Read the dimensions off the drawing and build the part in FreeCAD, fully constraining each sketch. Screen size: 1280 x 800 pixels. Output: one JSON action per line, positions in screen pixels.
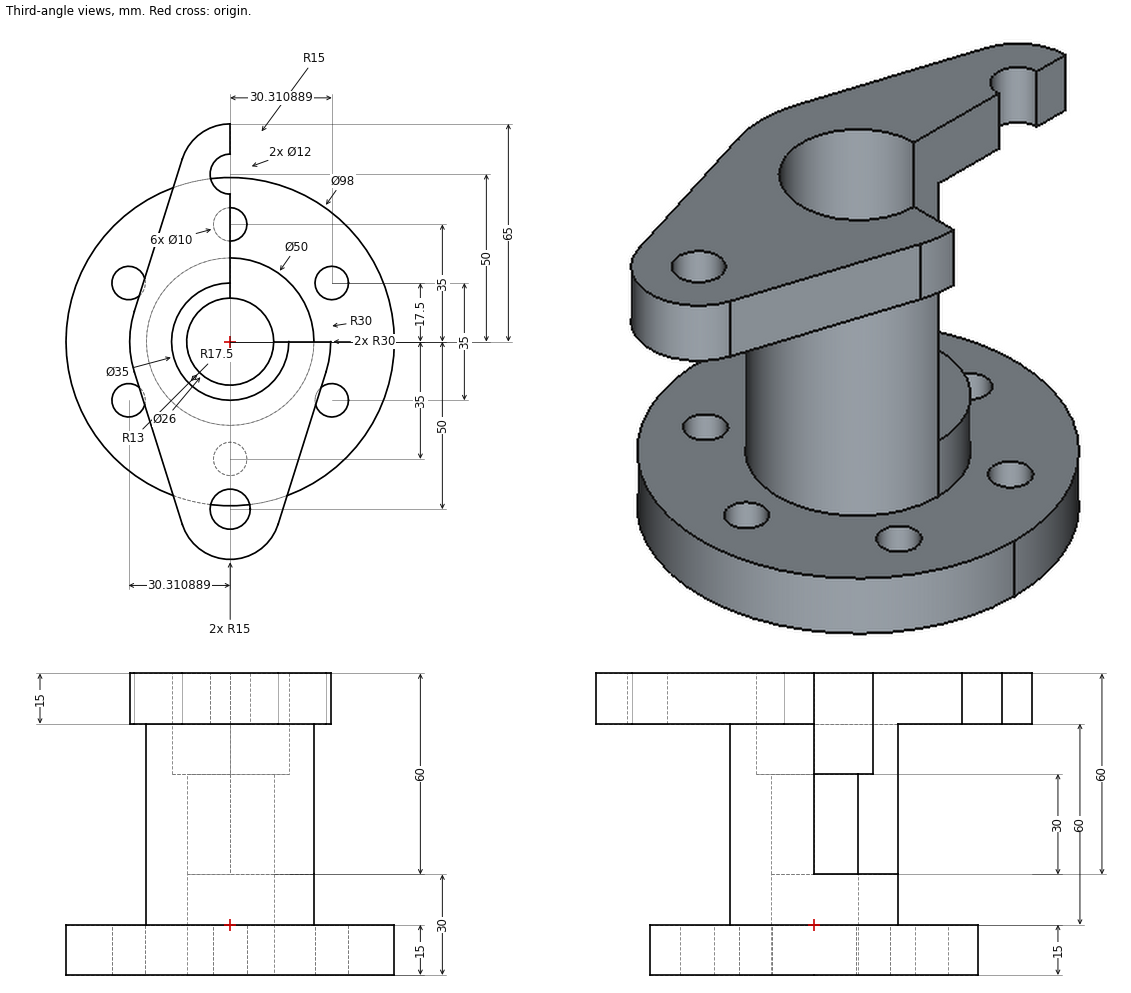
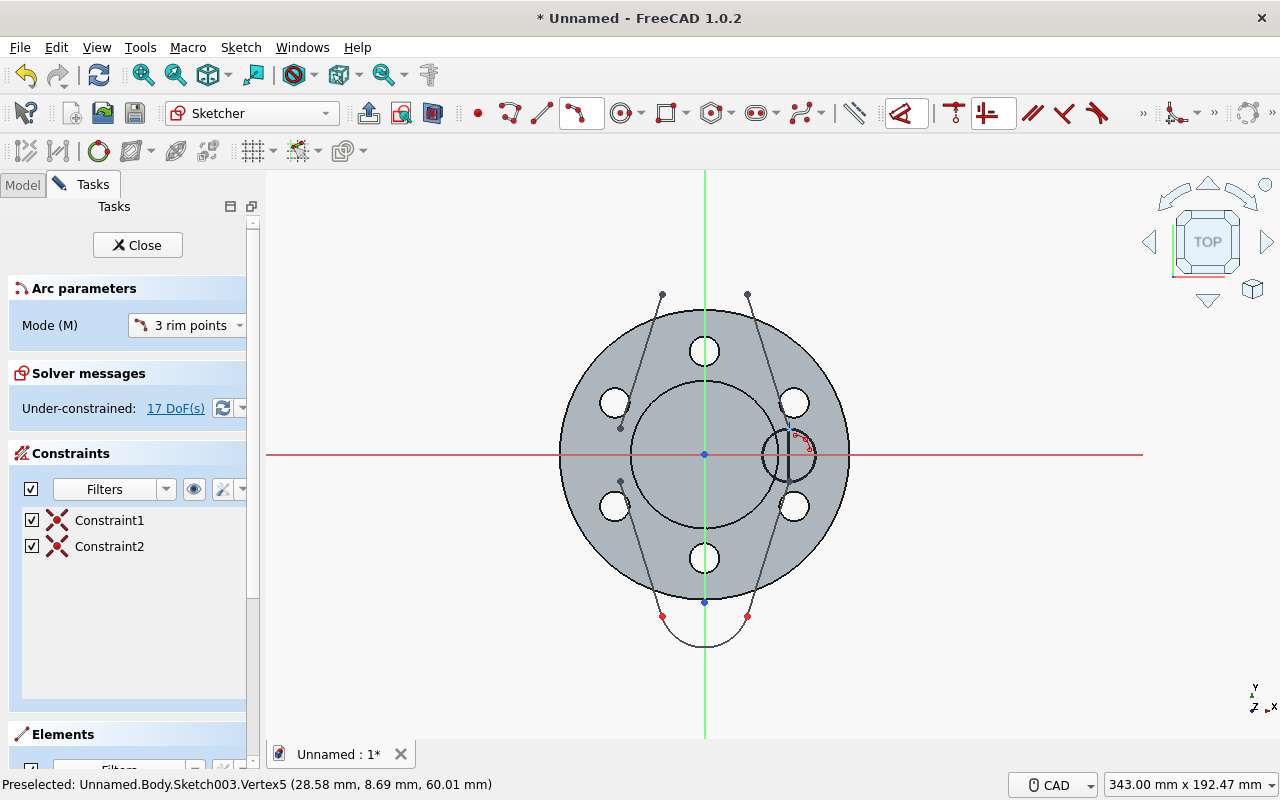
{"action": "scroll", "coordinate": [793, 460], "scroll_direction": "up", "scroll_amount": 7}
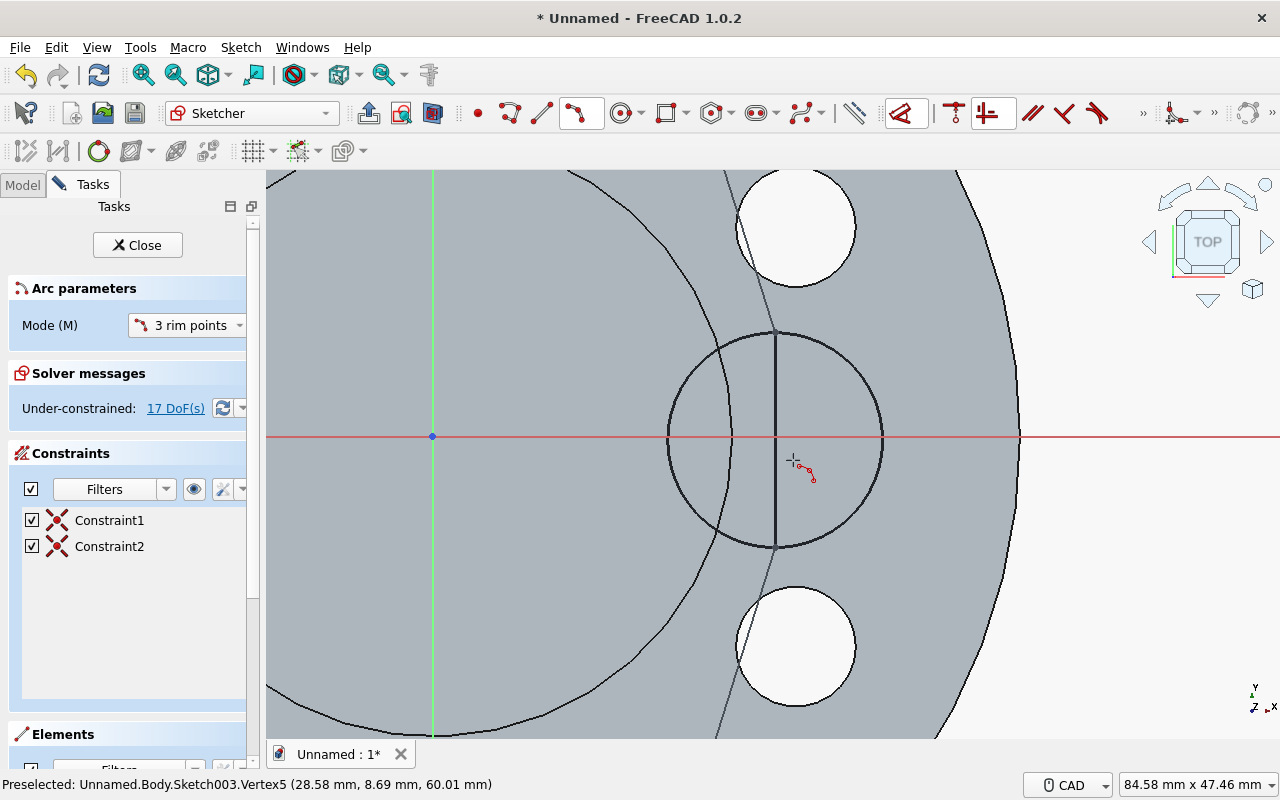
{"action": "left_click", "coordinate": [792, 459]}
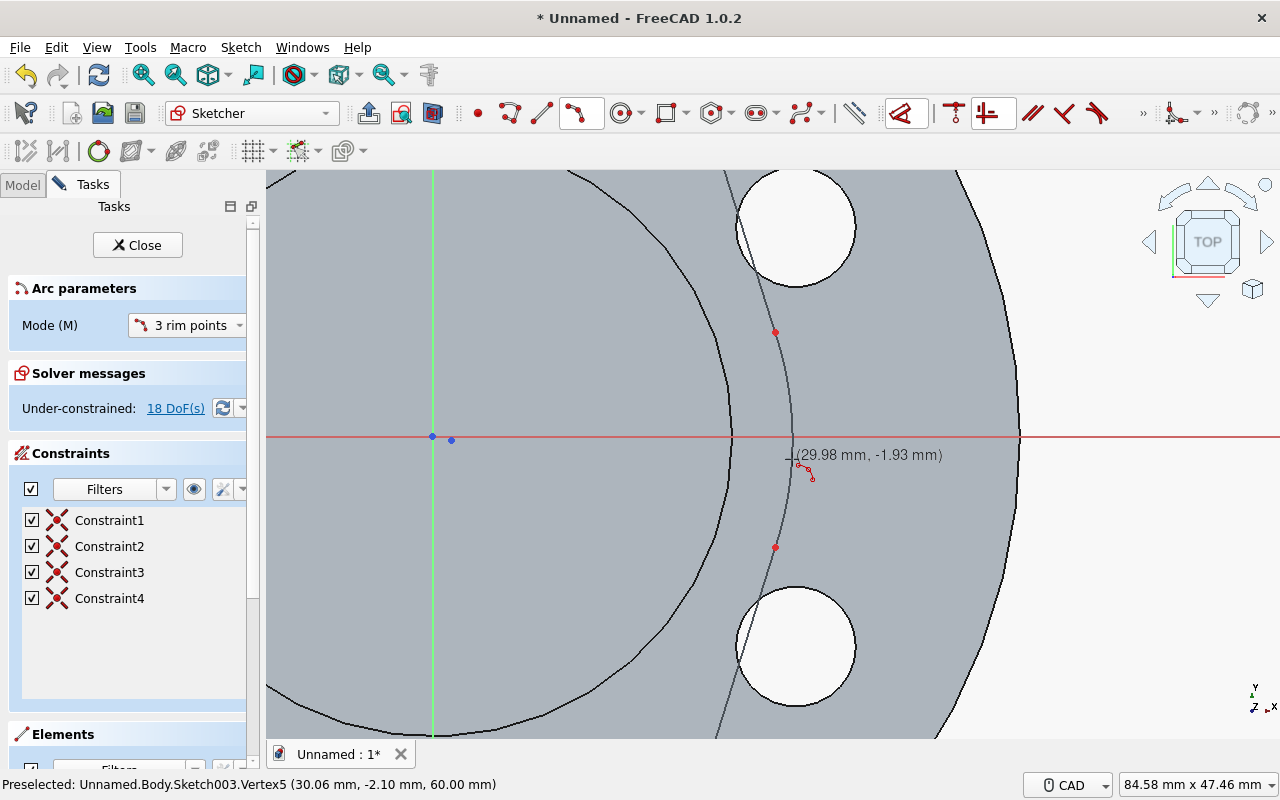
{"action": "scroll", "coordinate": [794, 460], "scroll_direction": "down", "scroll_amount": 7}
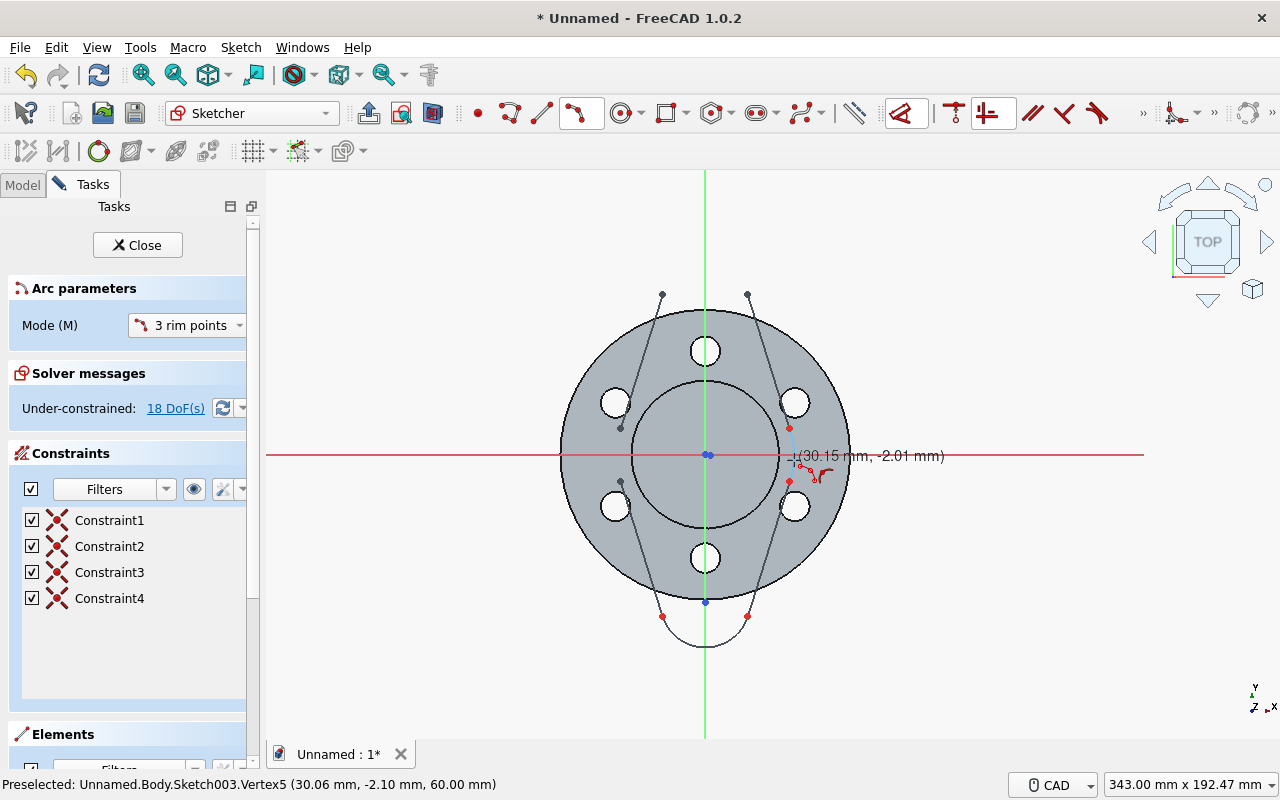
{"action": "left_click", "coordinate": [748, 295]}
{"action": "left_click", "coordinate": [663, 295]}
{"action": "left_click", "coordinate": [727, 268]}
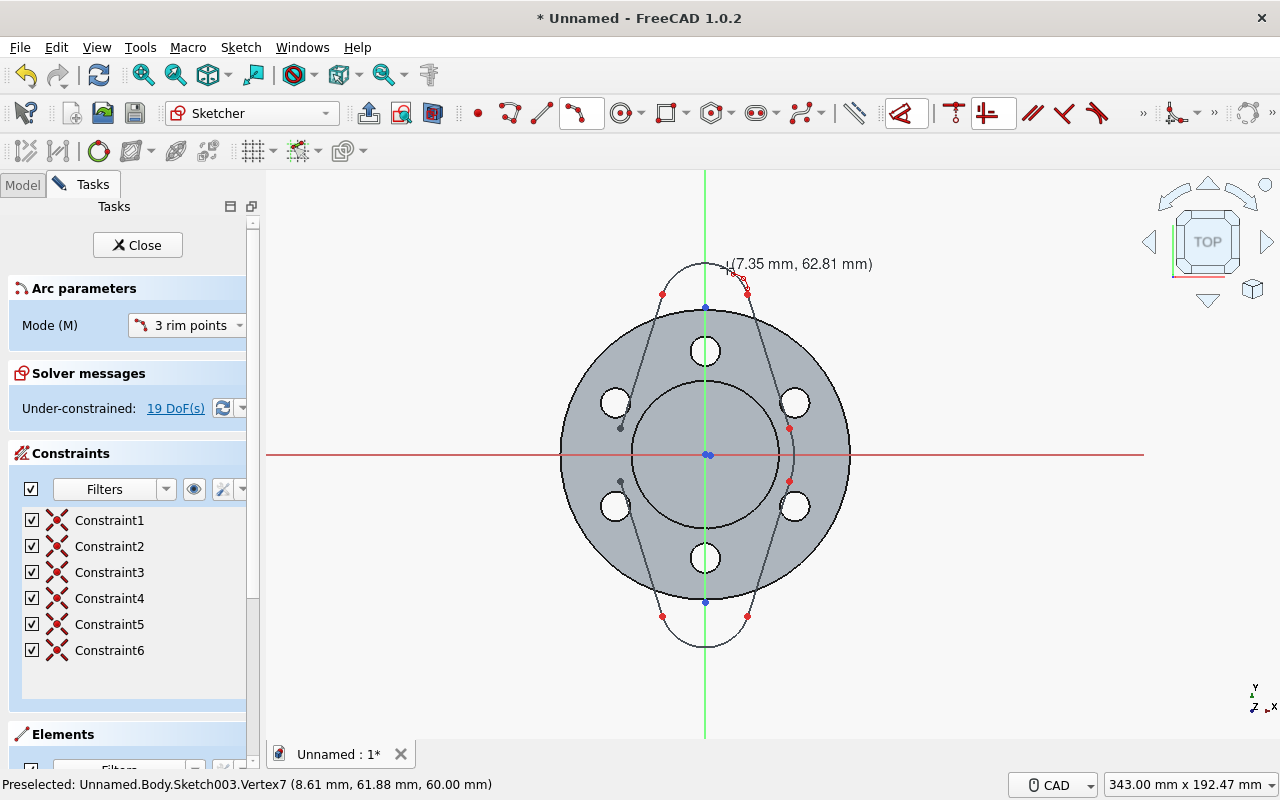
{"action": "left_click", "coordinate": [621, 429]}
{"action": "left_click", "coordinate": [621, 482]}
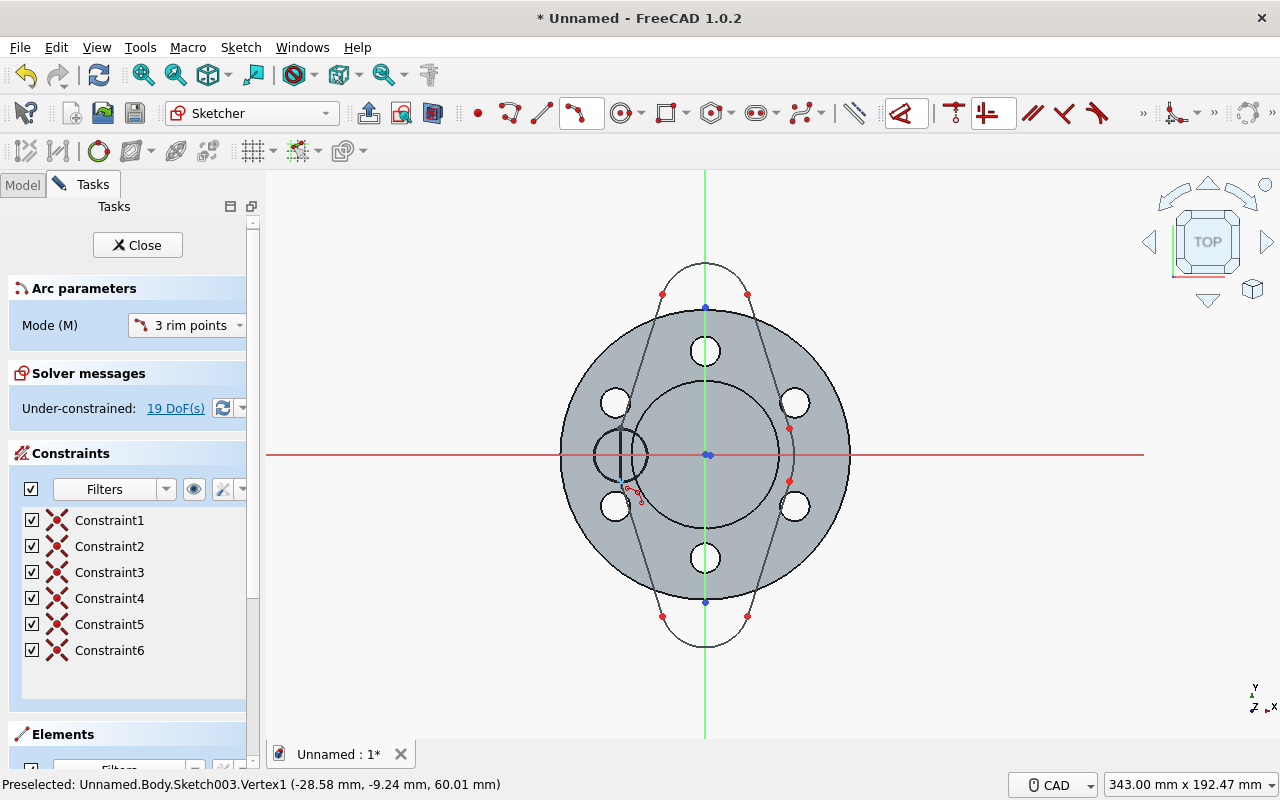
{"action": "scroll", "coordinate": [617, 449], "scroll_direction": "up", "scroll_amount": 7}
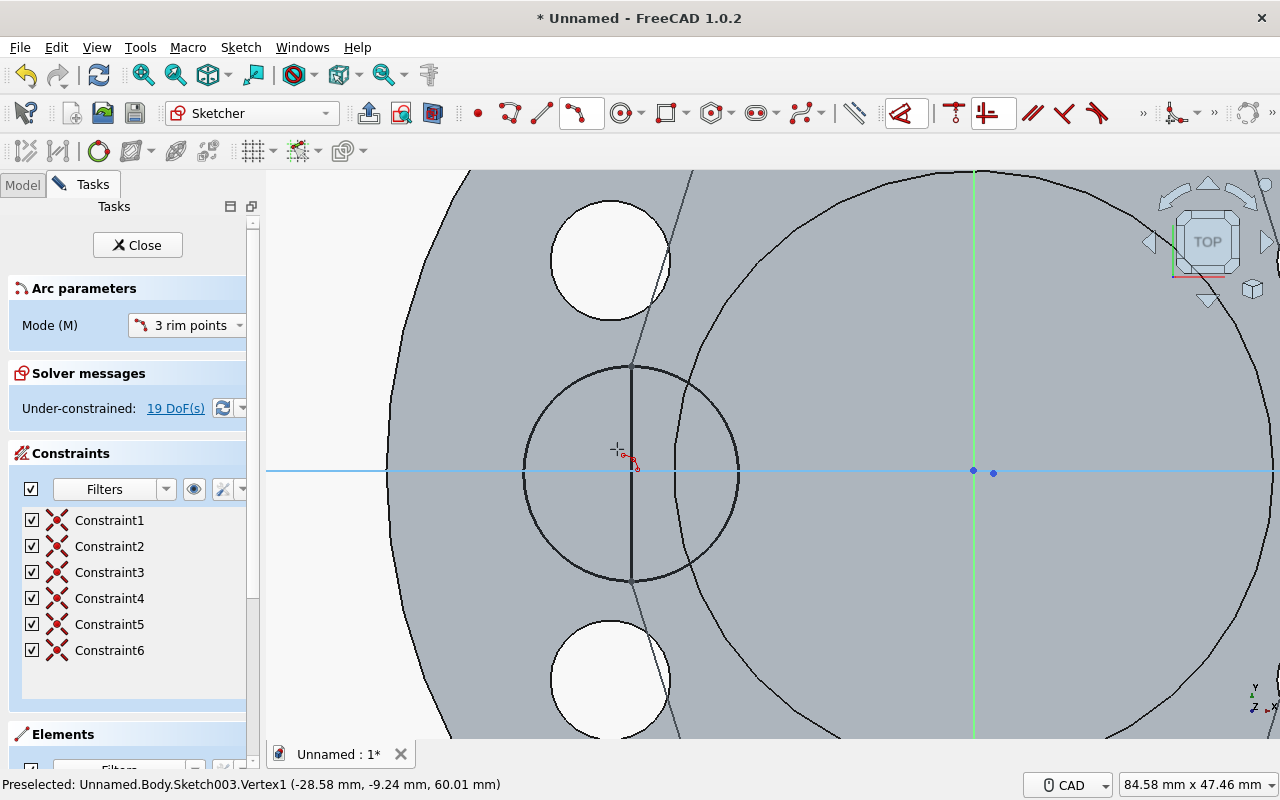
{"action": "left_click", "coordinate": [615, 449]}
{"action": "key", "text": "Escape"}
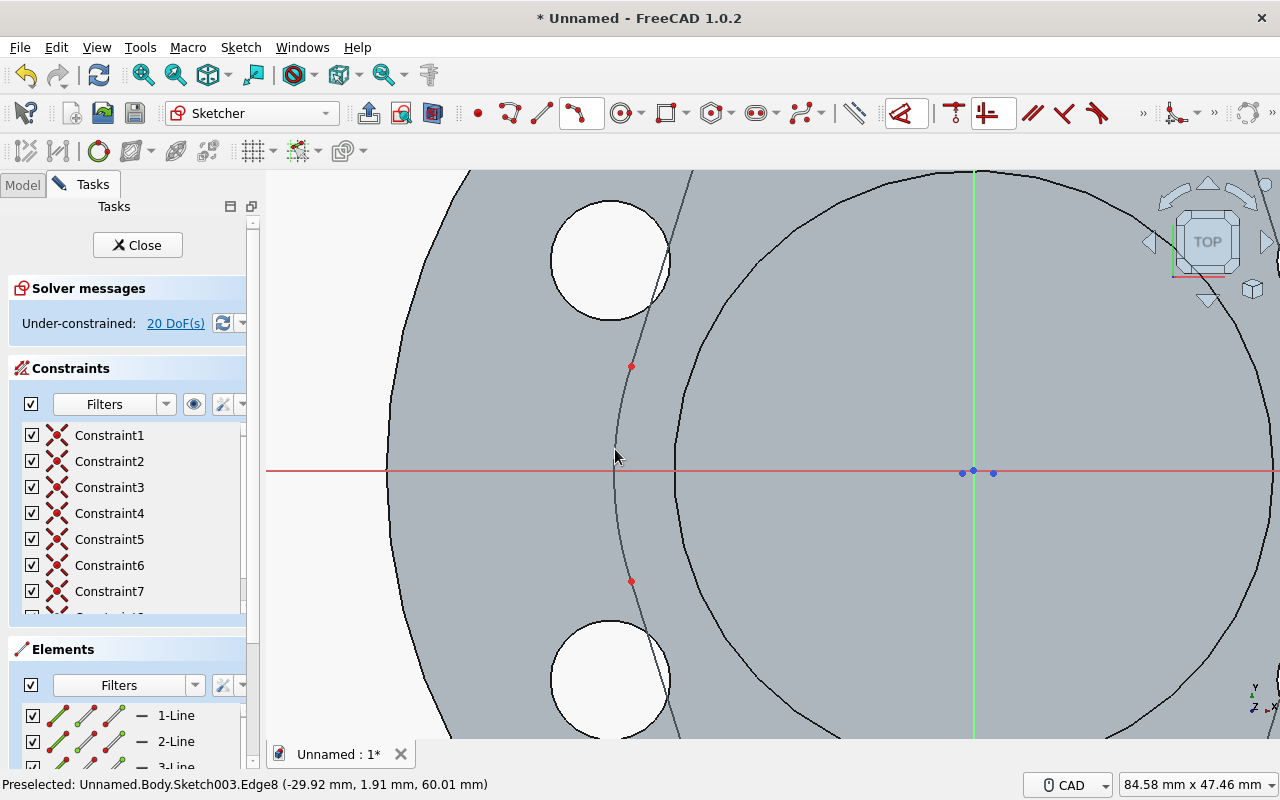
{"action": "scroll", "coordinate": [616, 449], "scroll_direction": "down", "scroll_amount": 7}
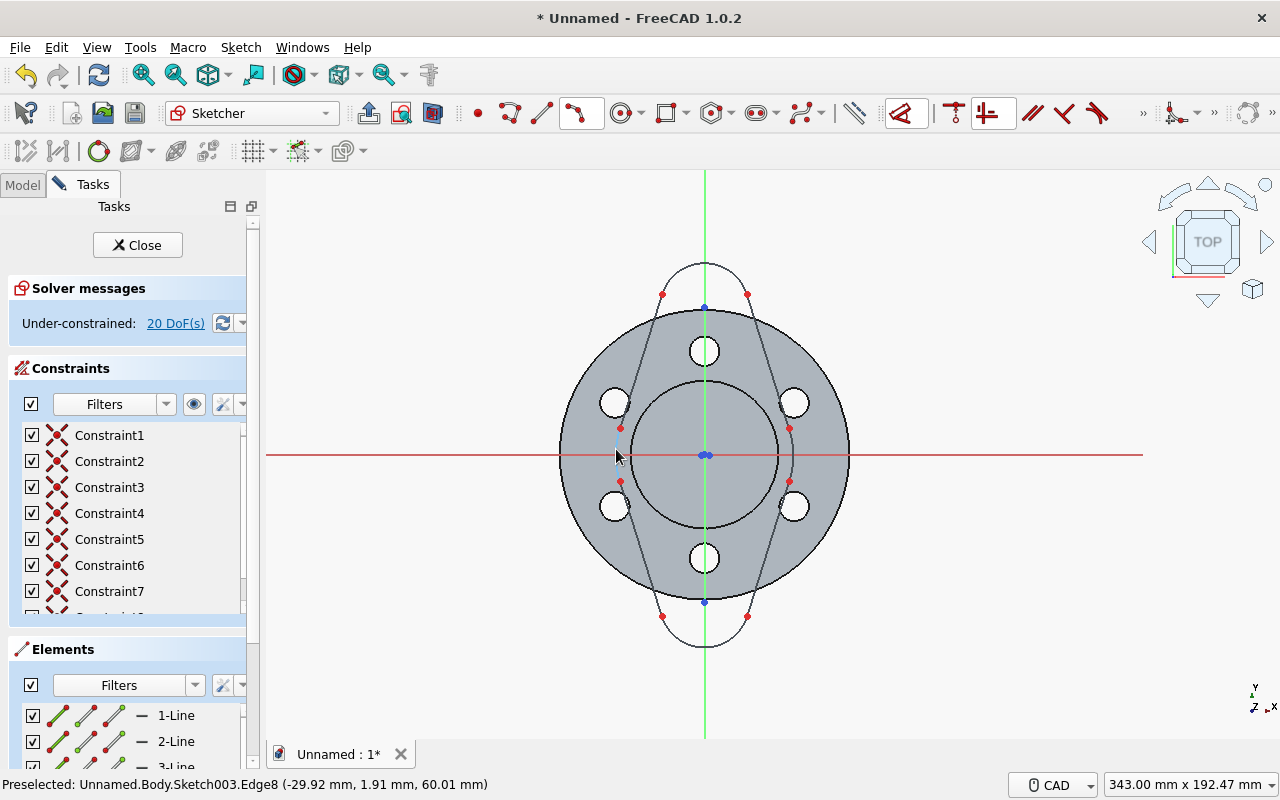
{"action": "left_click", "coordinate": [628, 509]}